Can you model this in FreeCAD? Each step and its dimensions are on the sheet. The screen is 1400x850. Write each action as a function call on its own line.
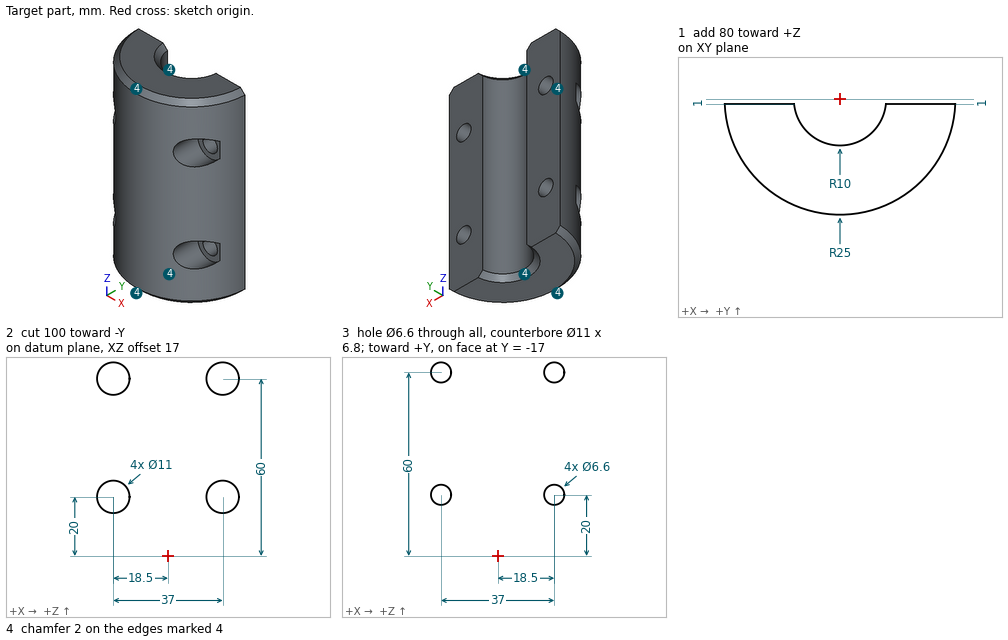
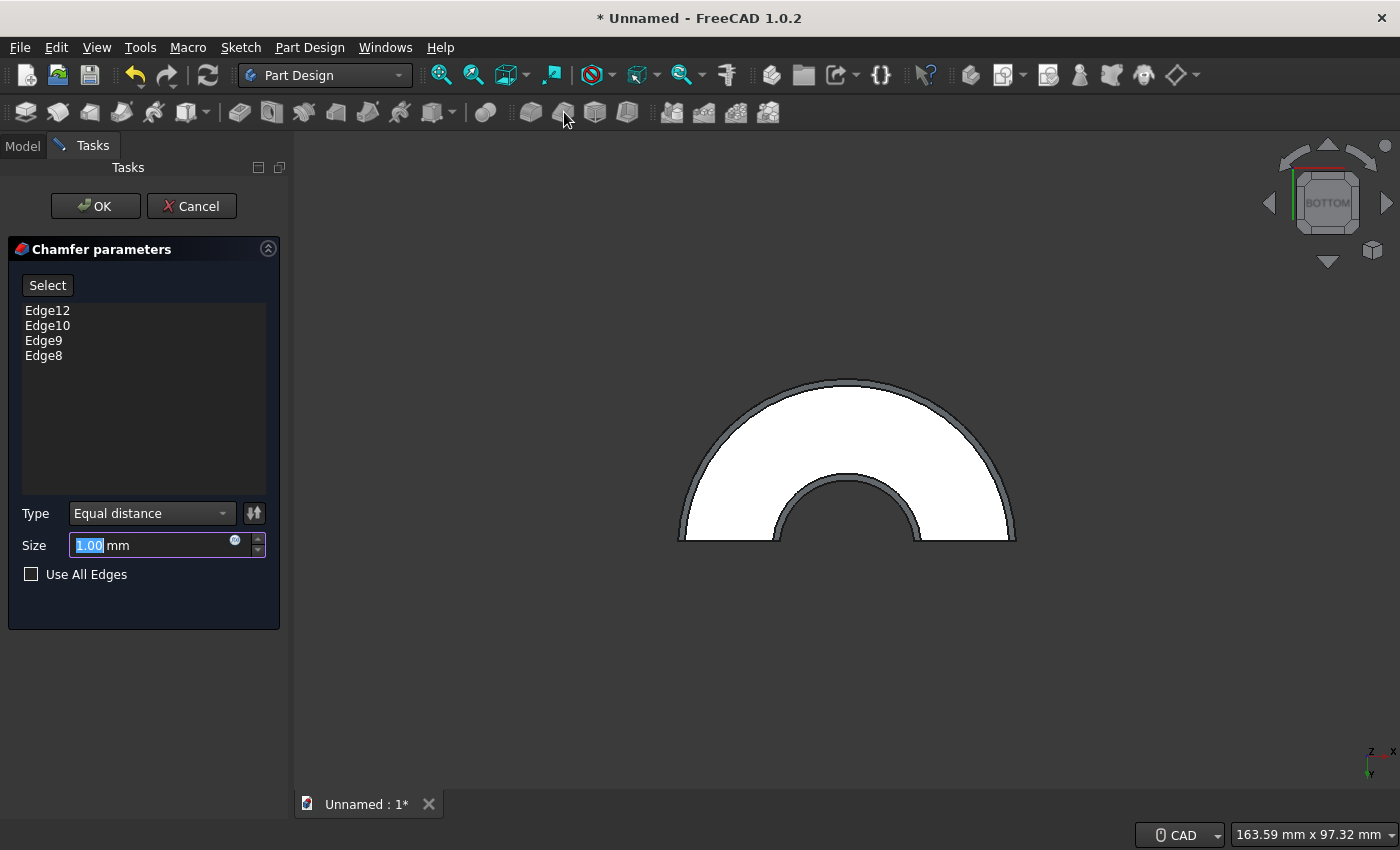
text(2)
key(Tab)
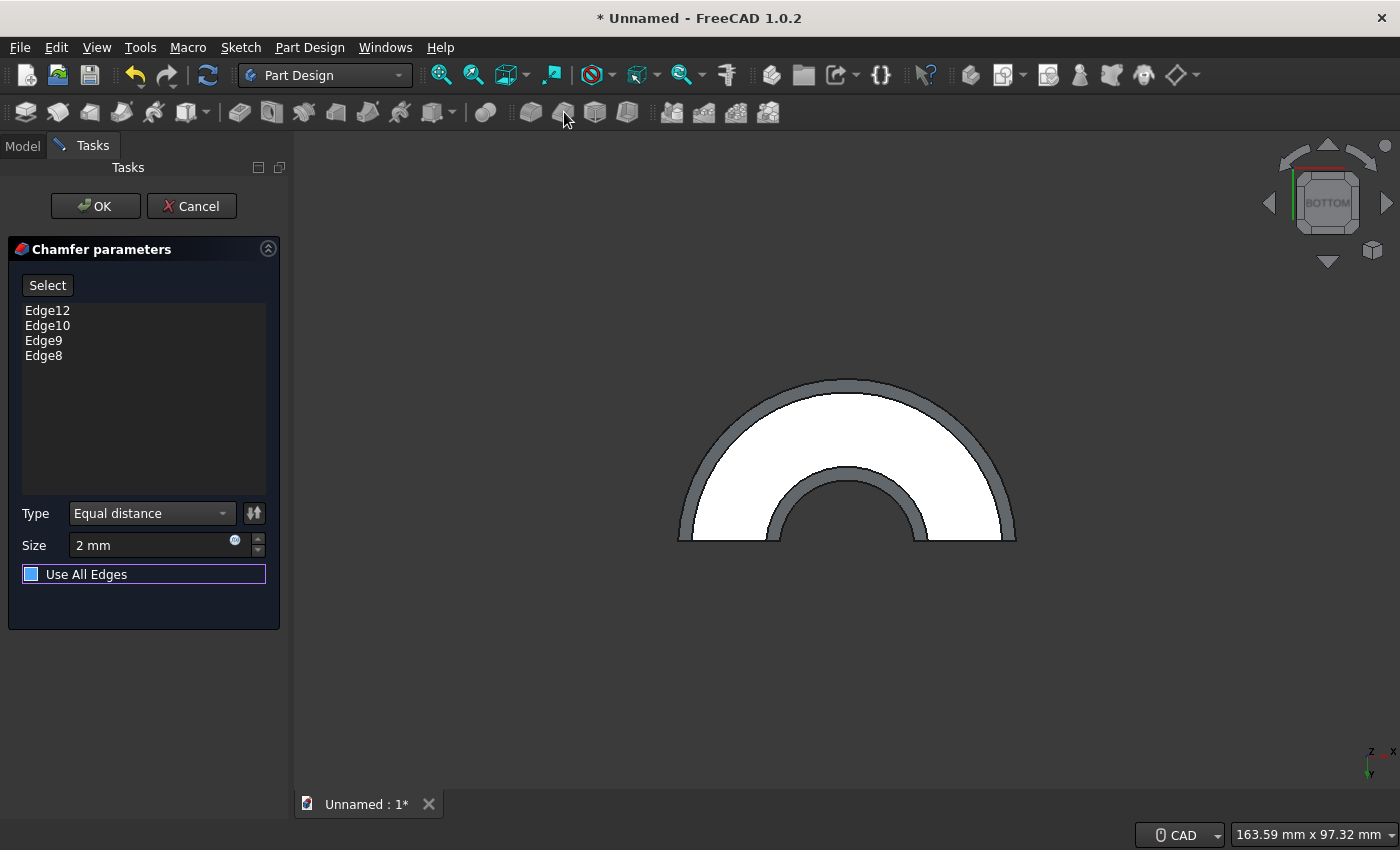
click(96, 206)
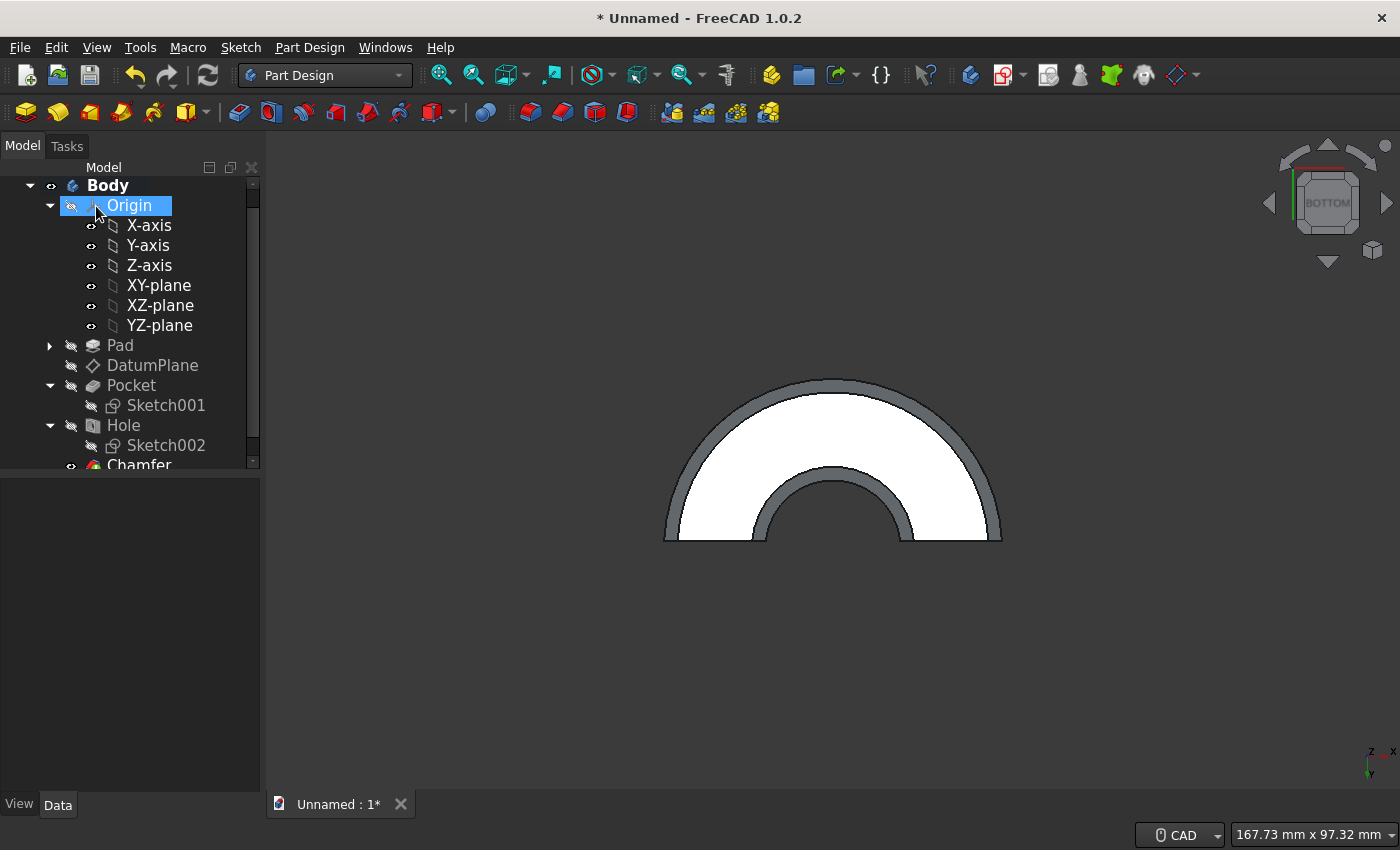
key(0)